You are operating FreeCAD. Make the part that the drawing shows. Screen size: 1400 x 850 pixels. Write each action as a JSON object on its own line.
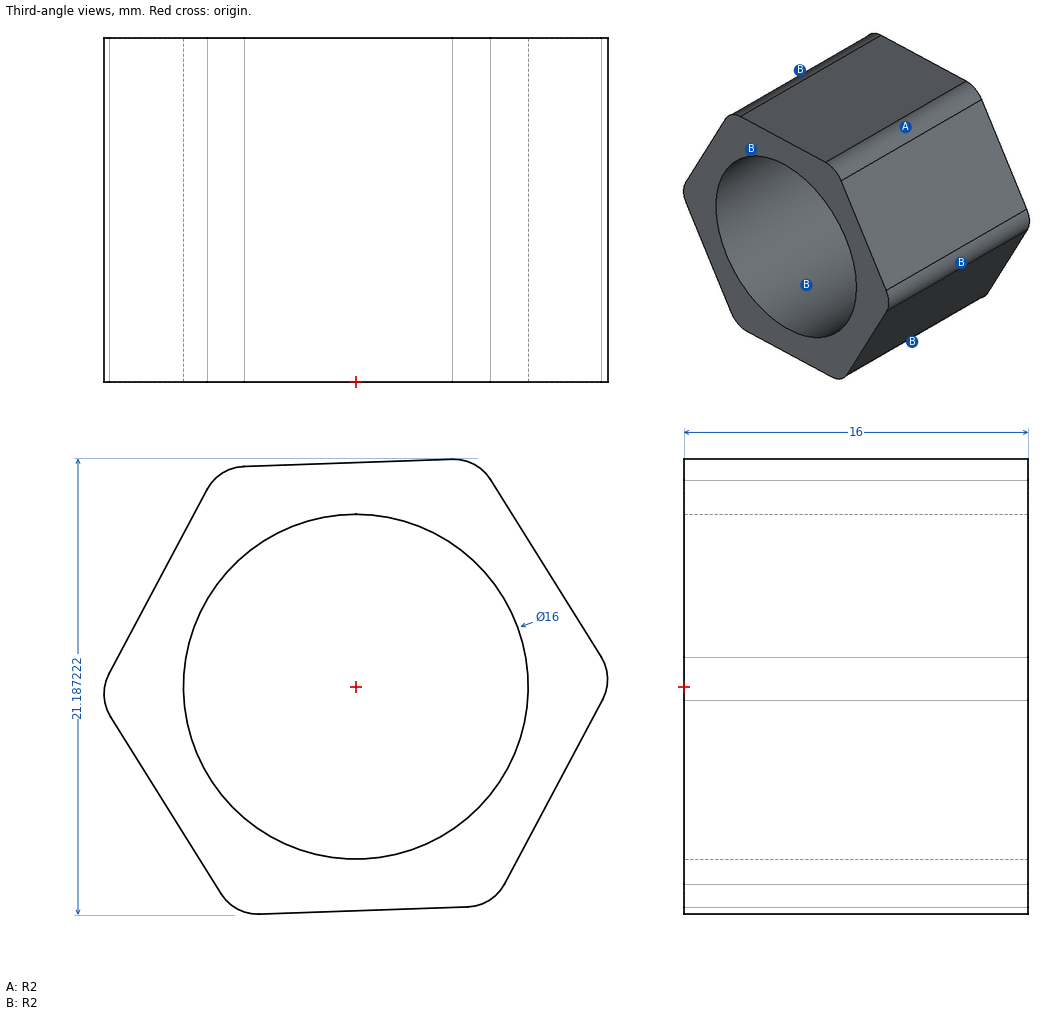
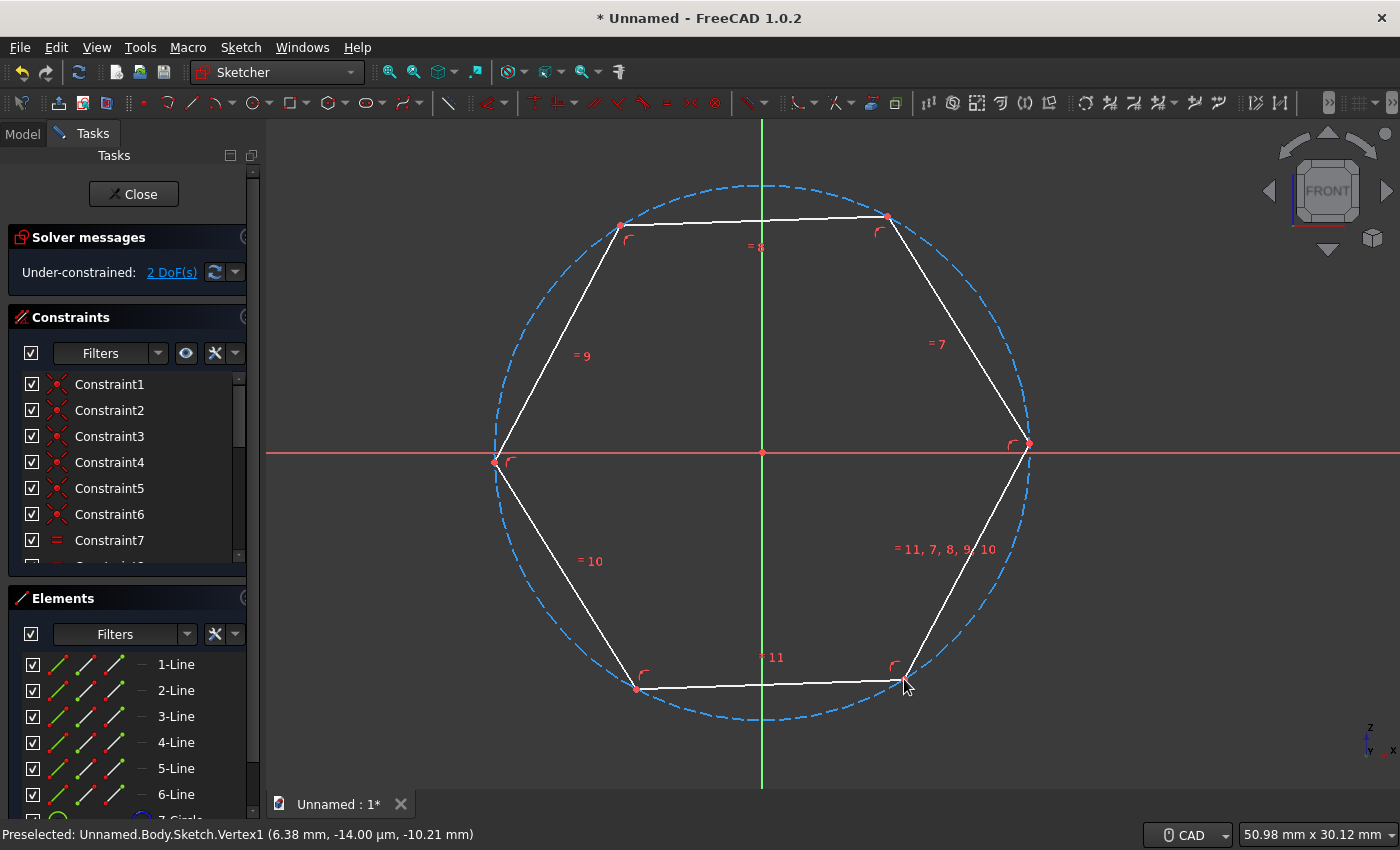
{"action": "left_click", "coordinate": [254, 104]}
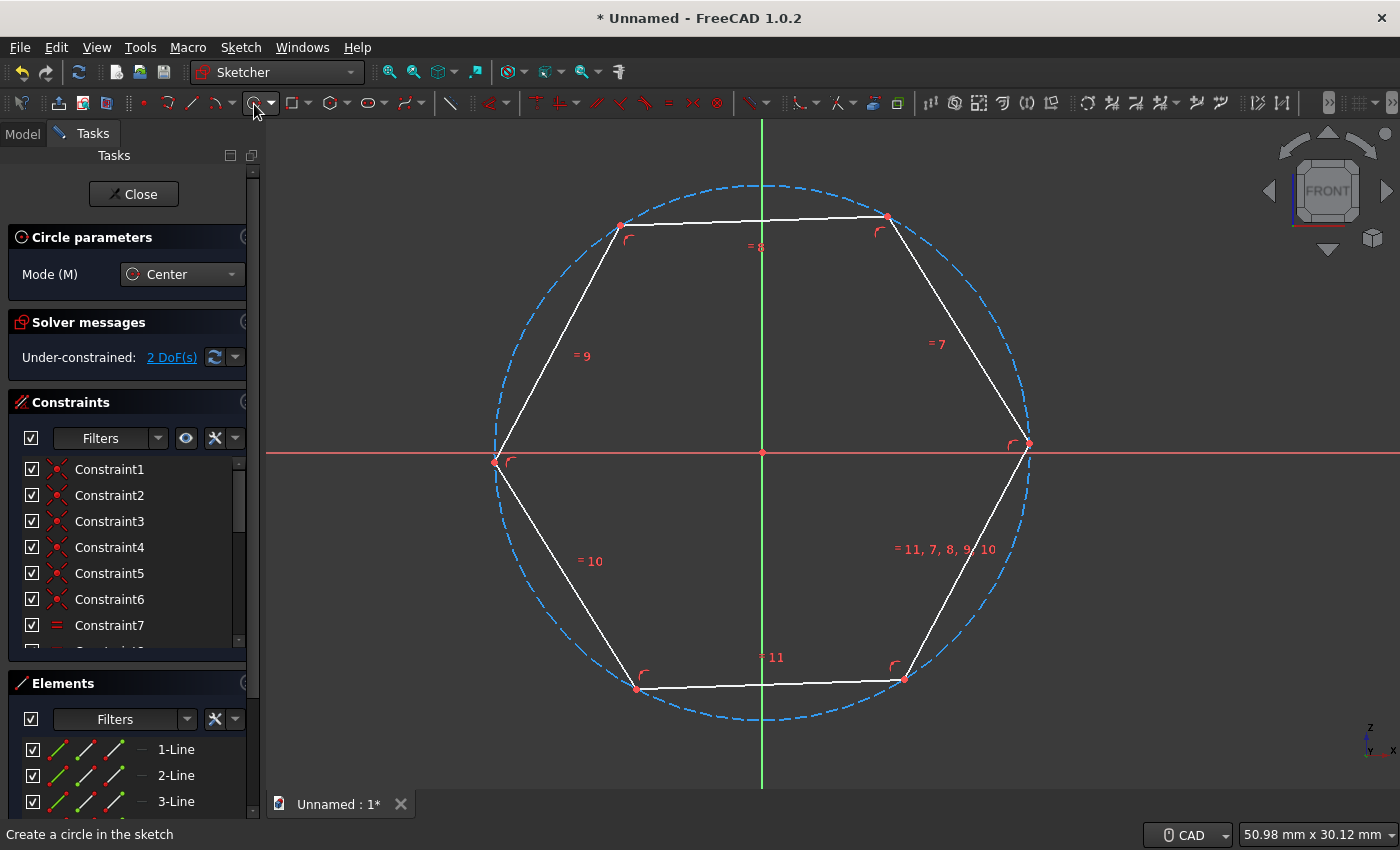
{"action": "left_click", "coordinate": [762, 453]}
{"action": "mouse_move", "coordinate": [888, 327]}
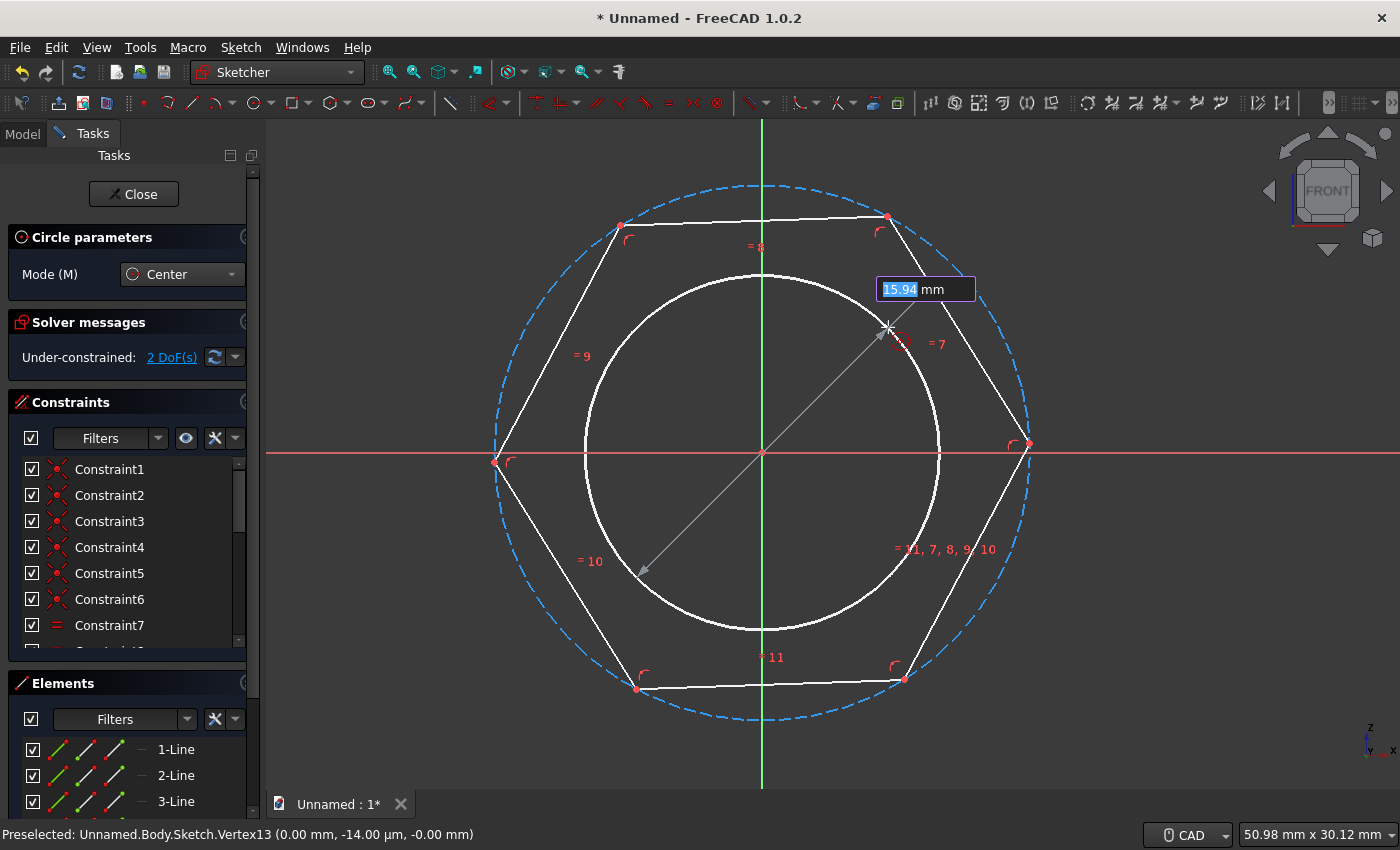
{"action": "type", "text": "16"}
{"action": "key", "text": "Return"}
{"action": "key", "text": "Escape"}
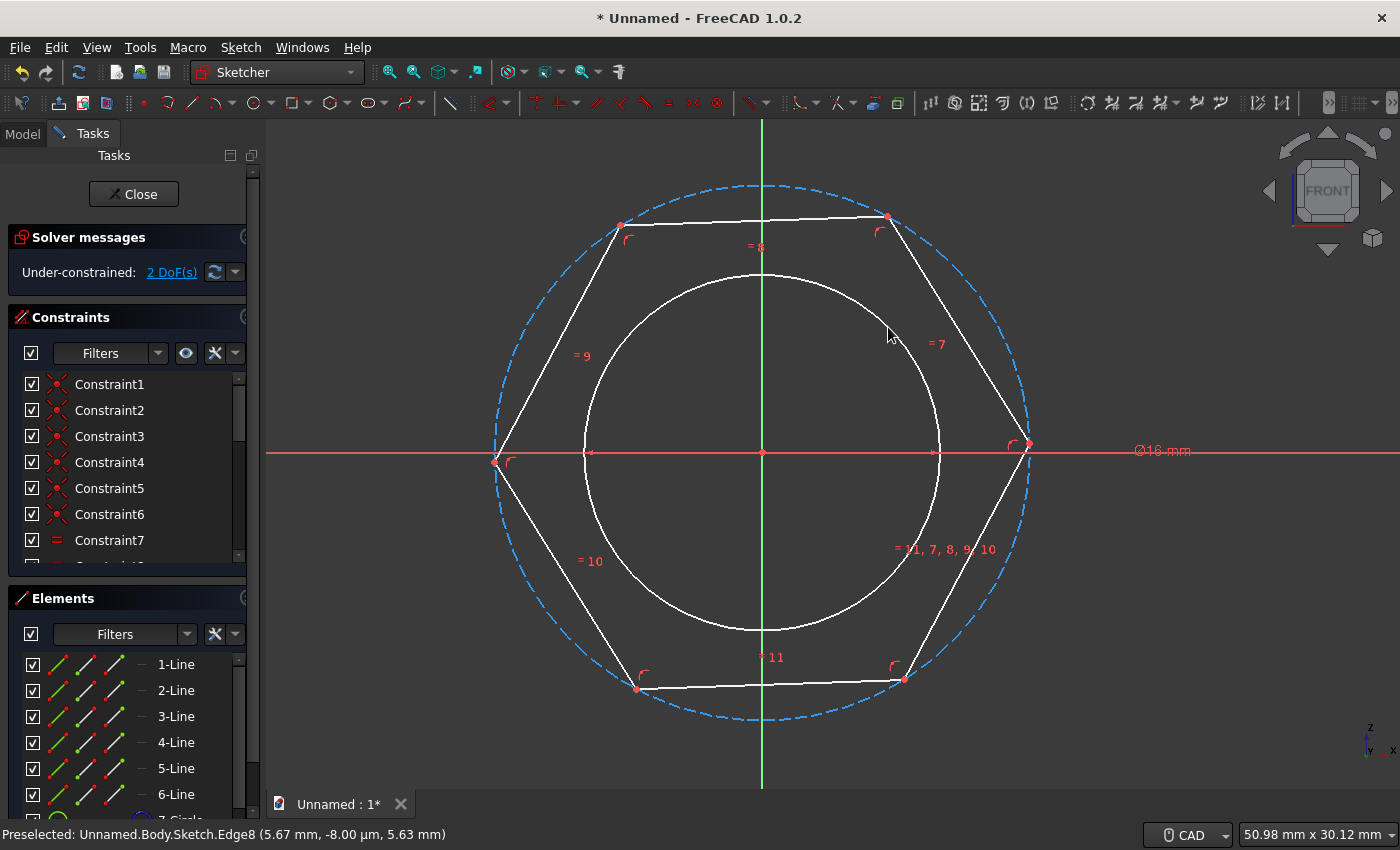
{"action": "left_click", "coordinate": [490, 104]}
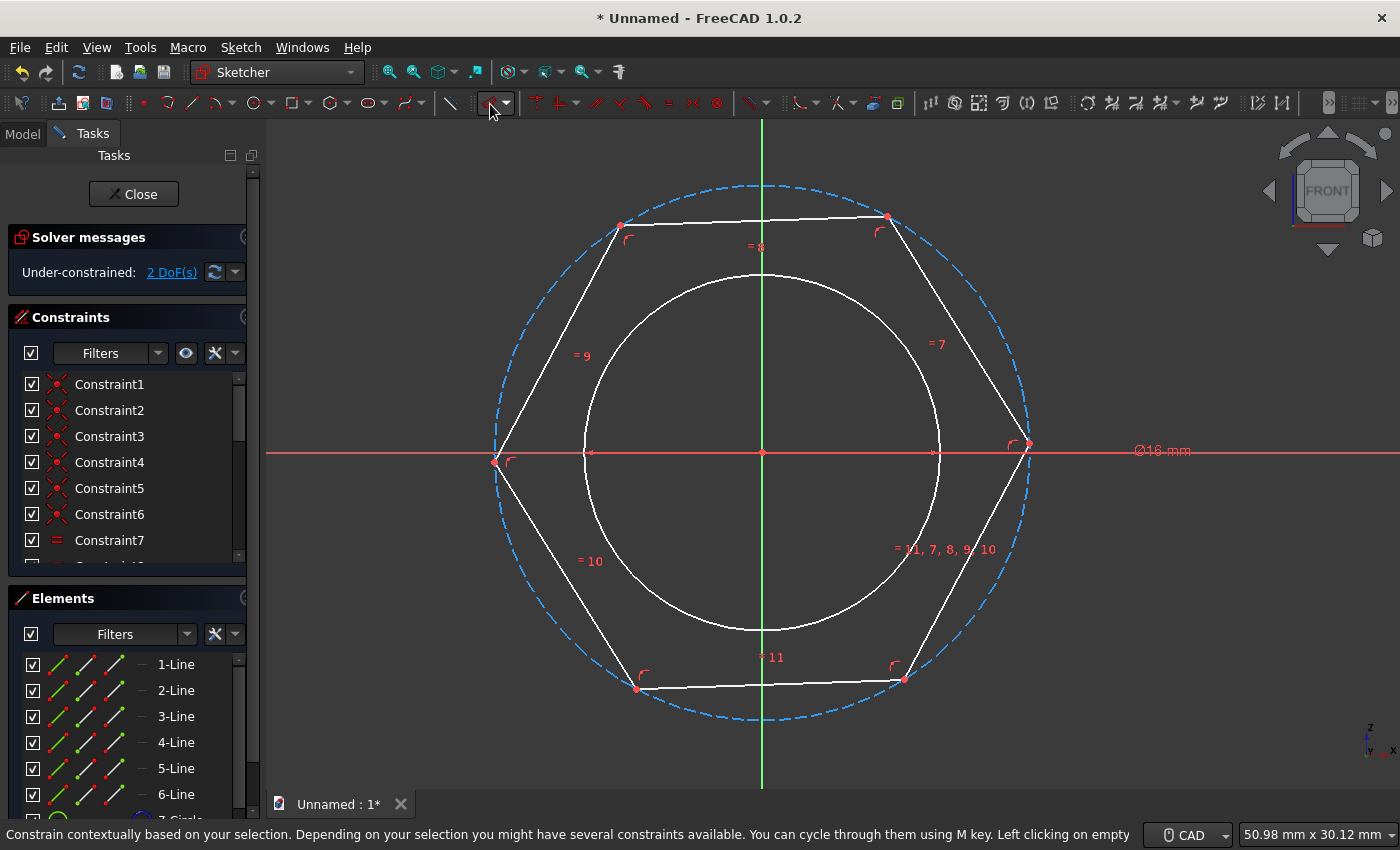
{"action": "left_click", "coordinate": [951, 263]}
{"action": "left_click", "coordinate": [974, 240]}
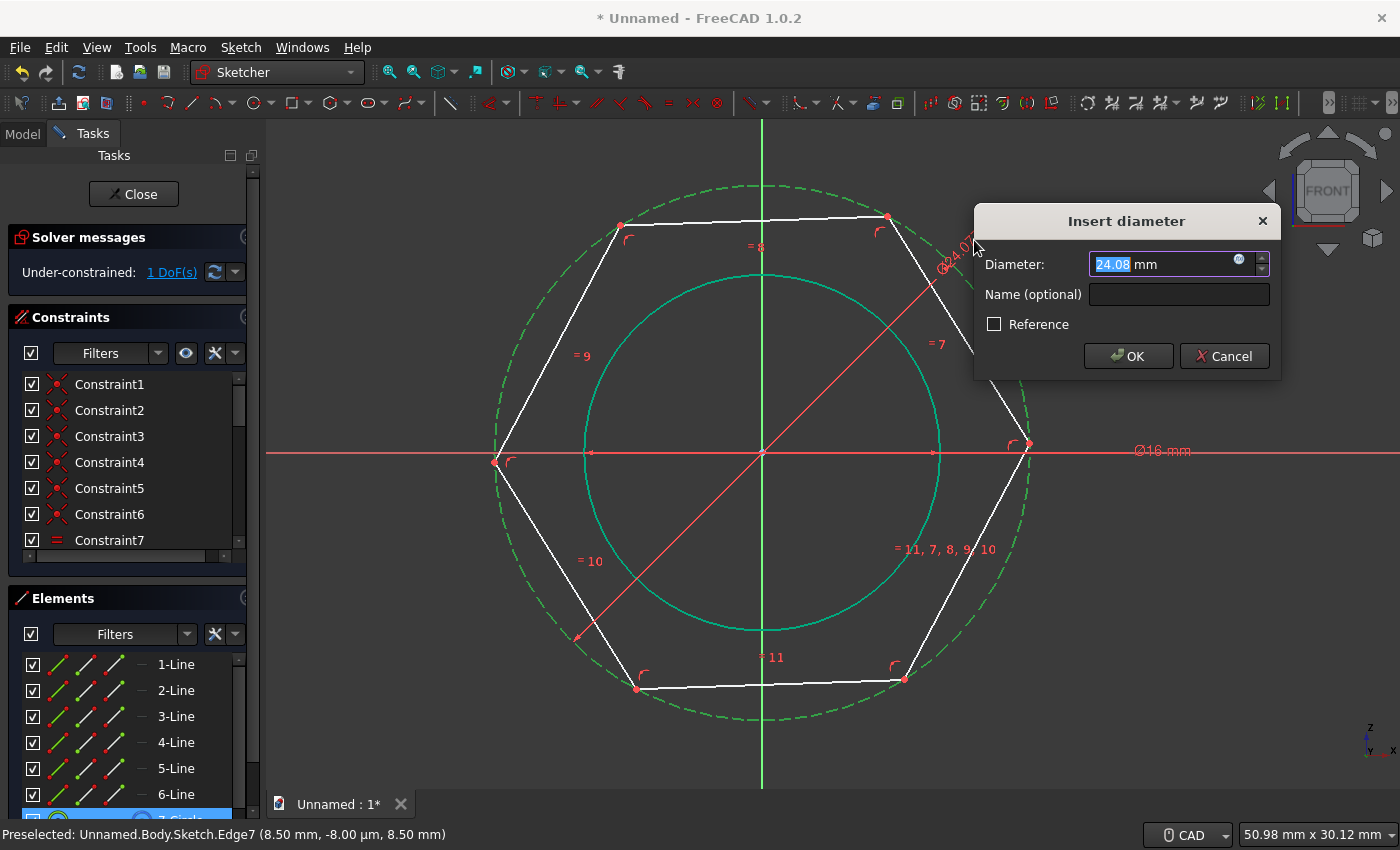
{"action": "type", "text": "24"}
{"action": "key", "text": "Return"}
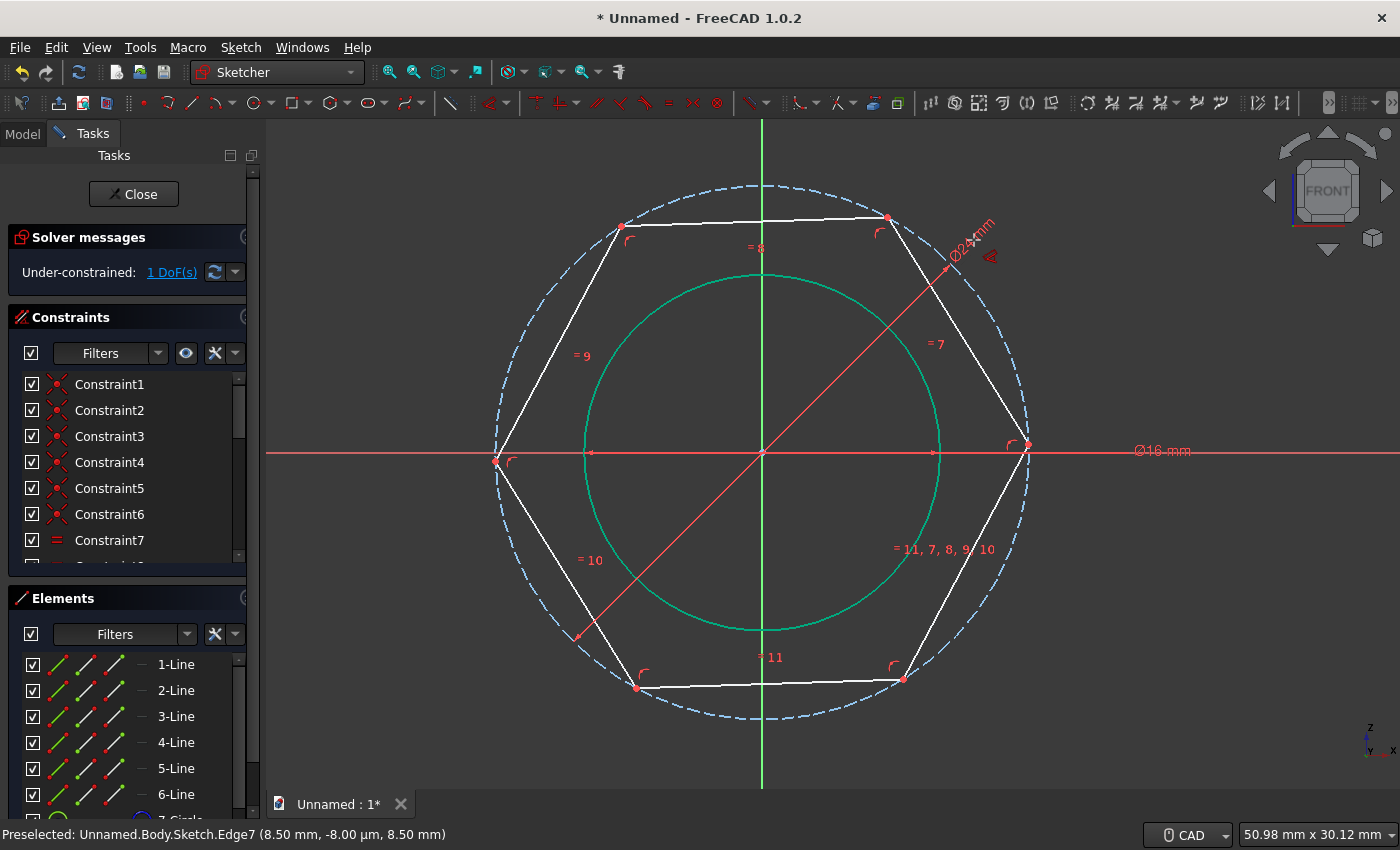
{"action": "left_click", "coordinate": [636, 688]}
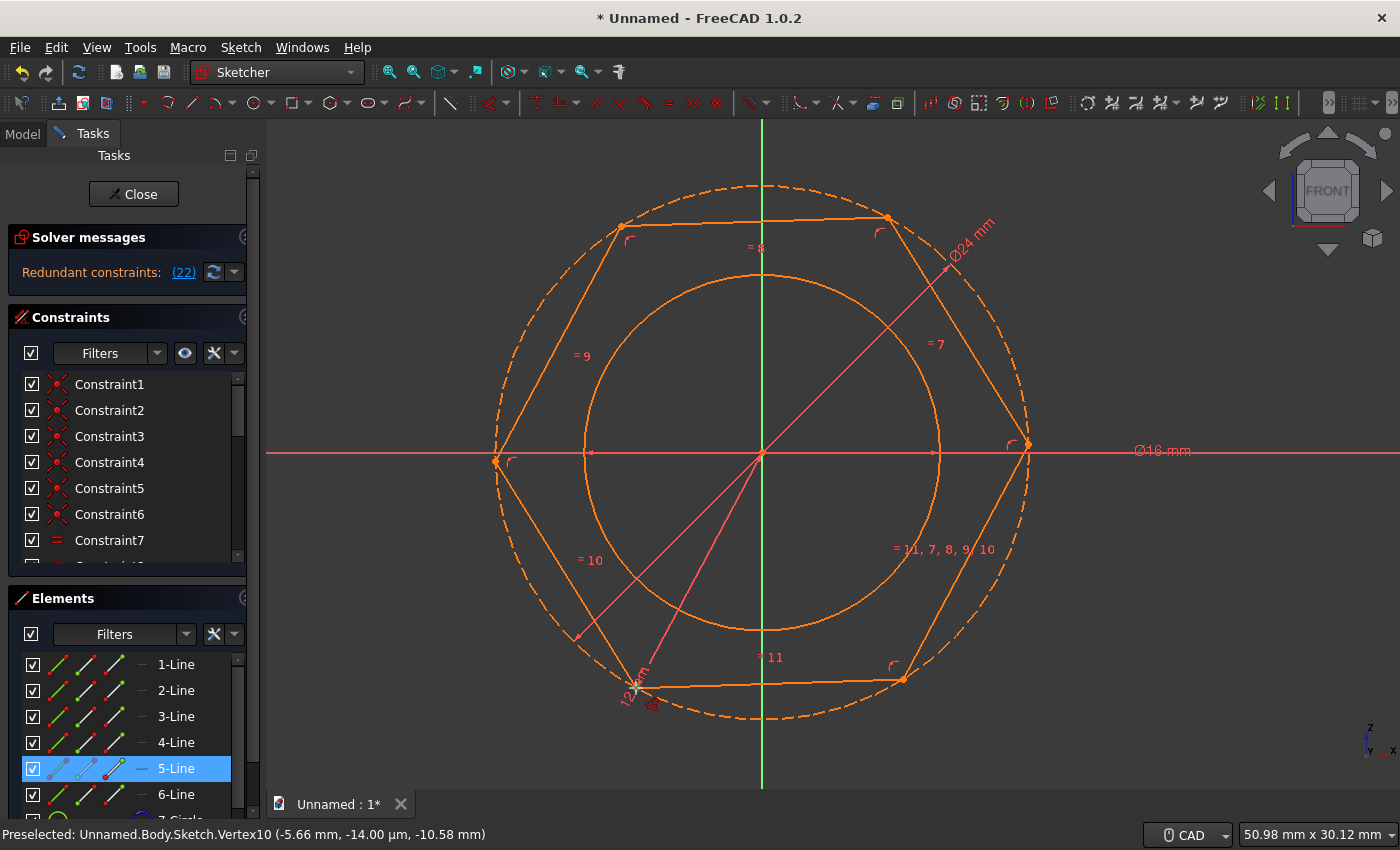
{"action": "left_click", "coordinate": [888, 217]}
{"action": "left_click", "coordinate": [922, 345]}